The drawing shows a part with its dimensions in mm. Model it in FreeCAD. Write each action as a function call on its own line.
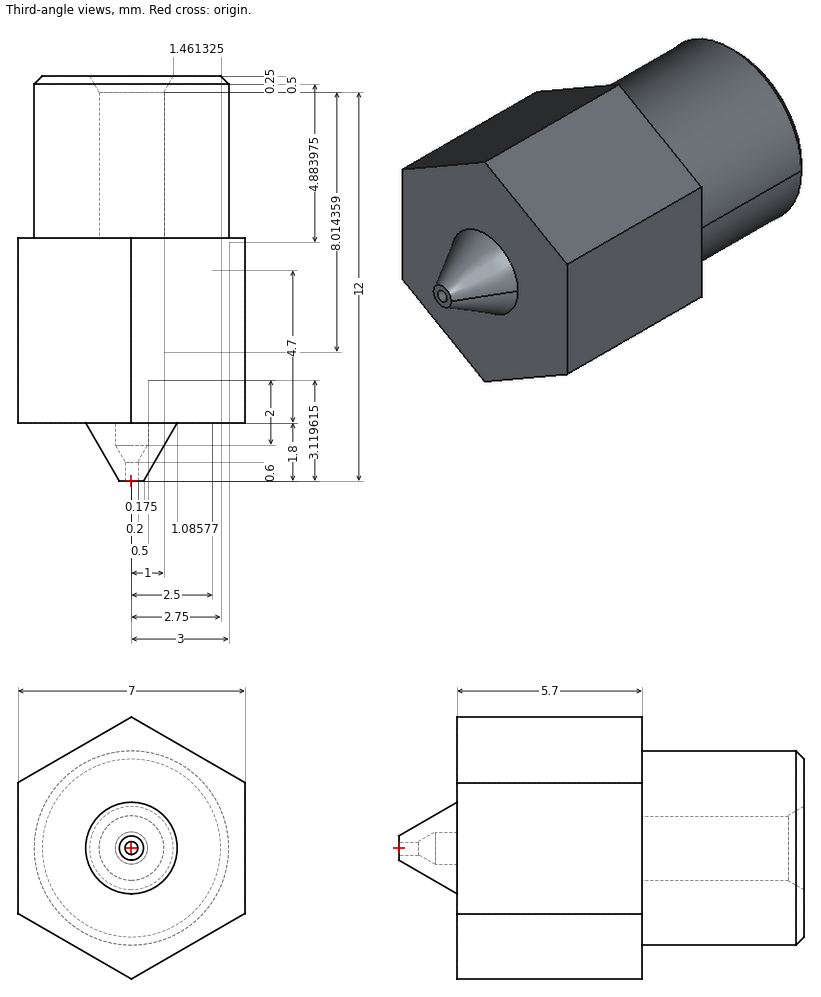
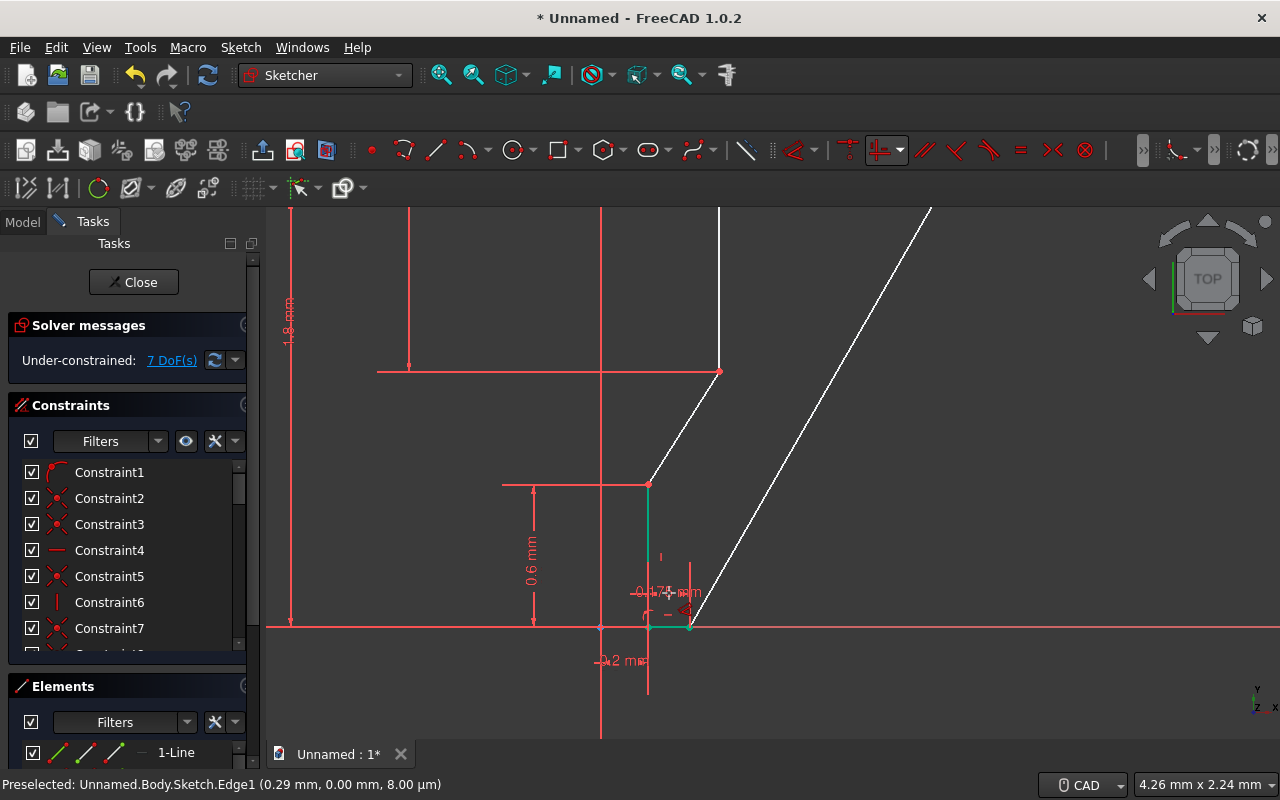
scroll(673, 639, down, 11)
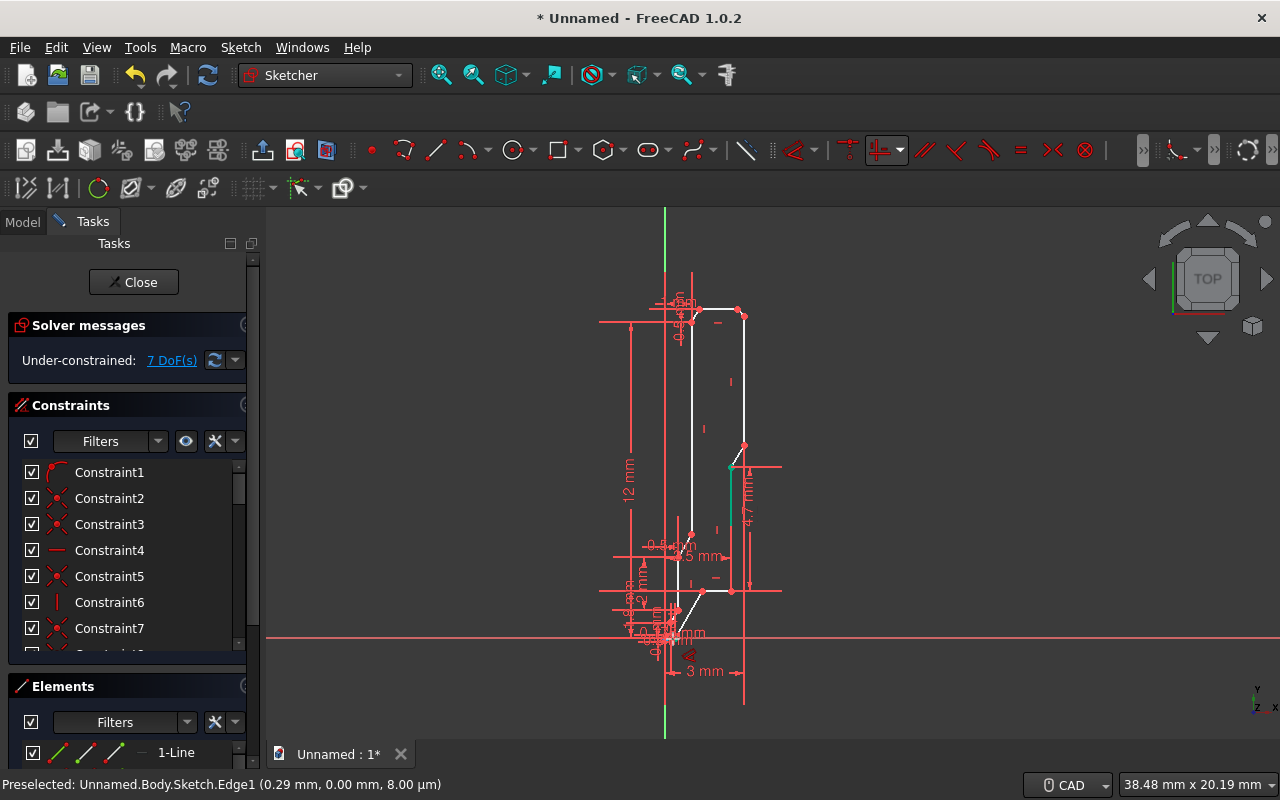
click(738, 309)
click(702, 275)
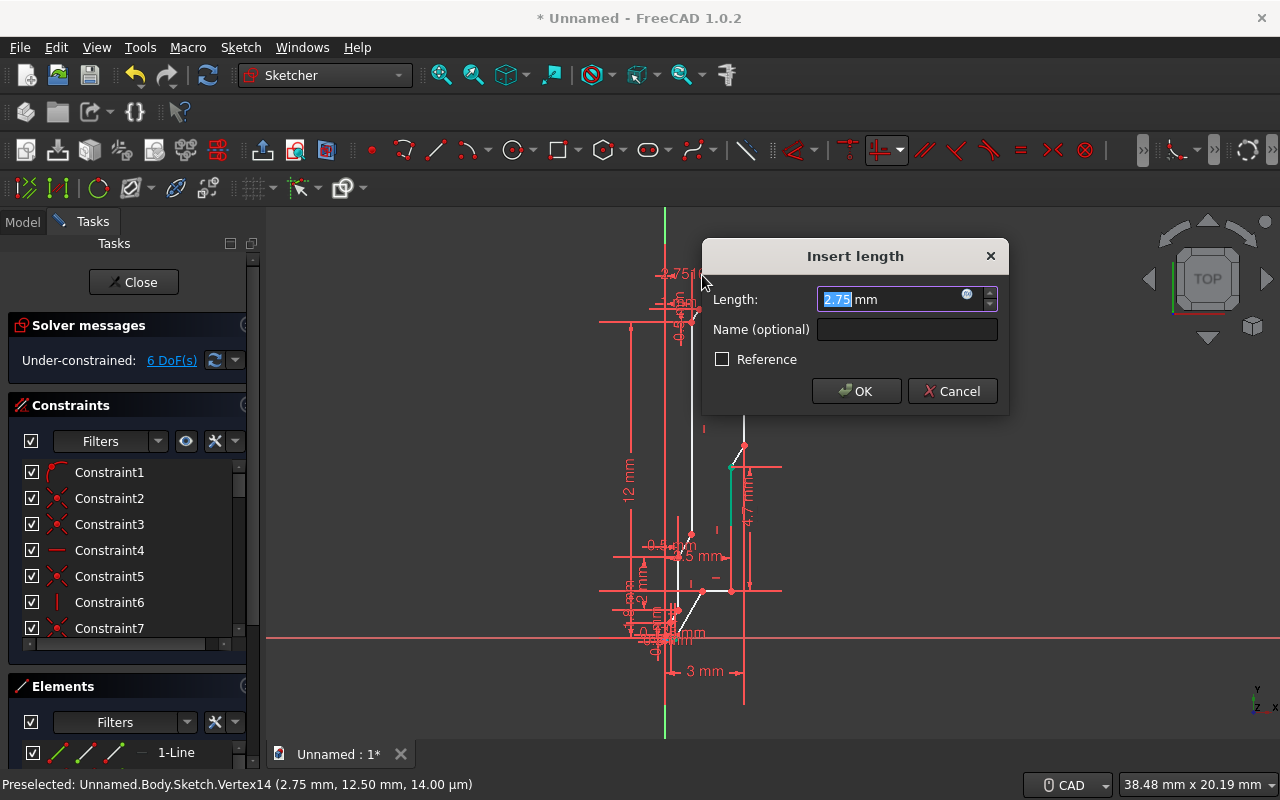
text(2.75)
key(Return)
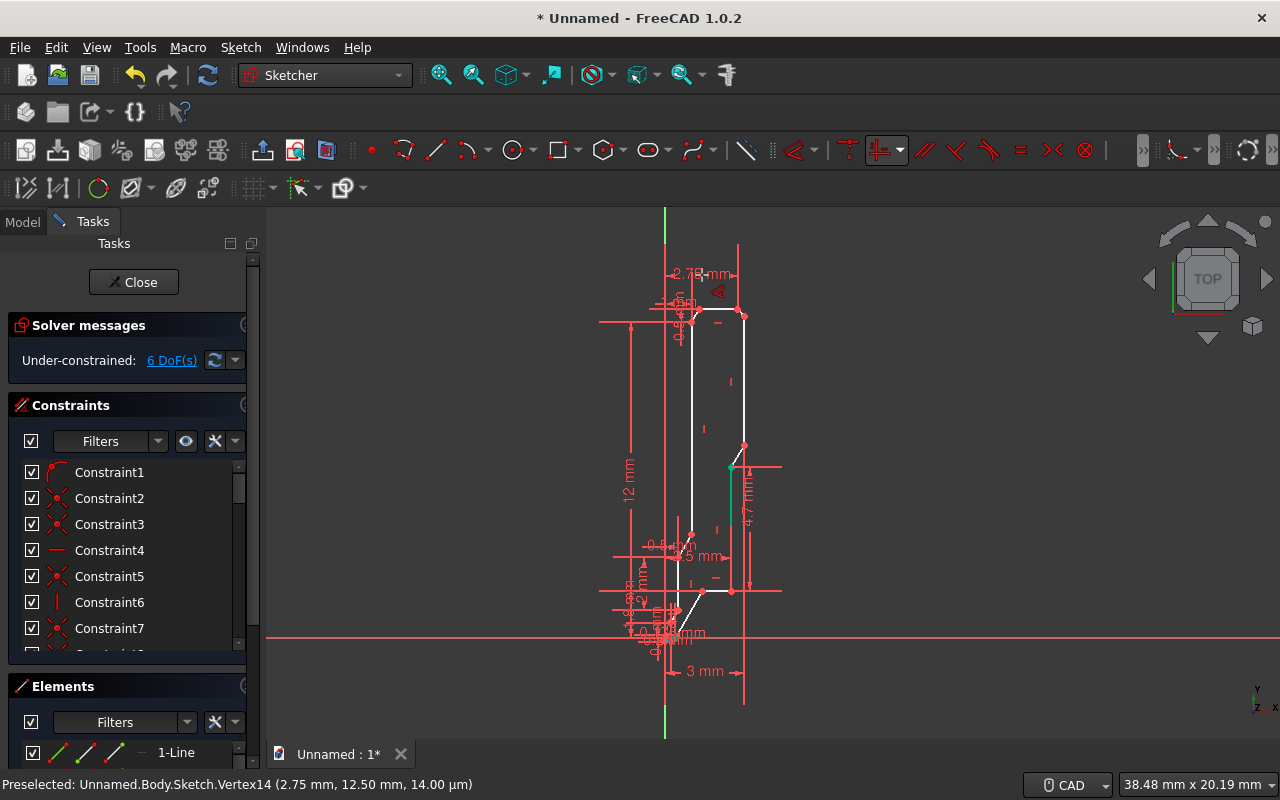
scroll(741, 313, up, 9)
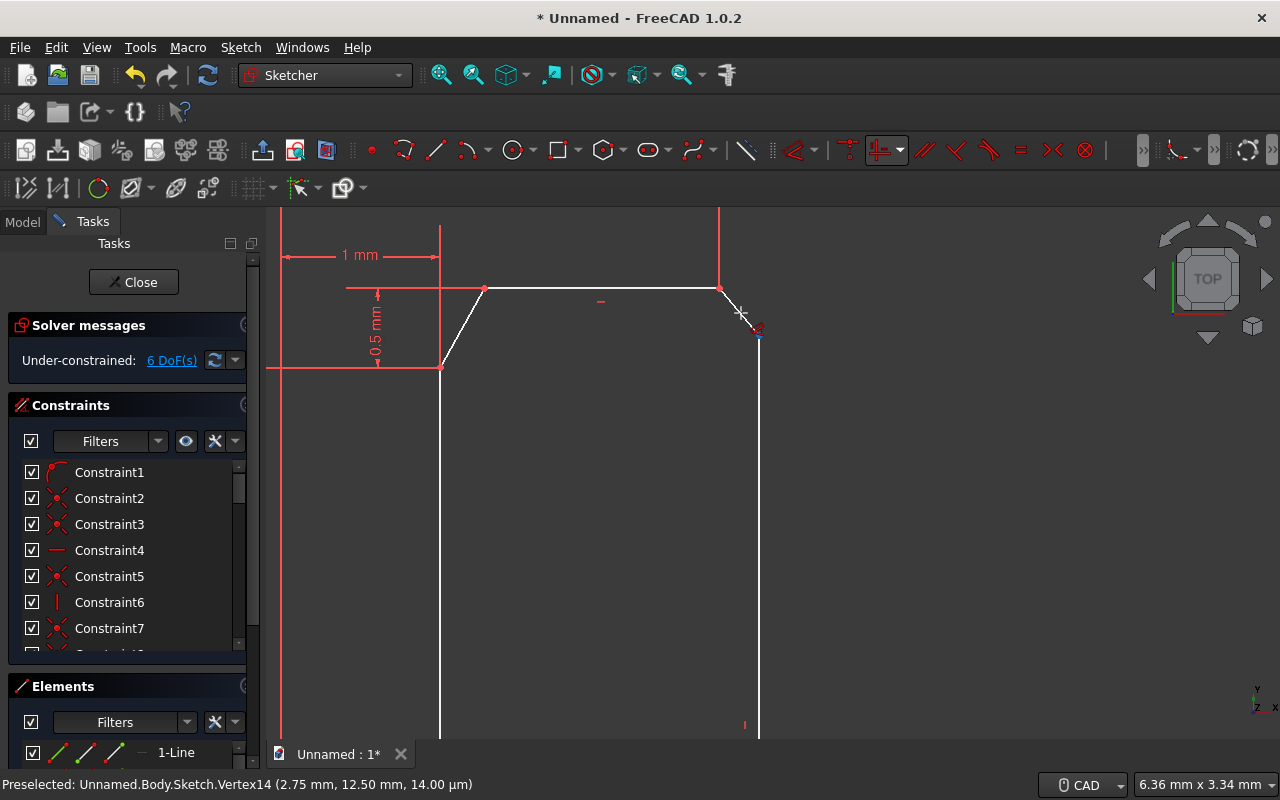
click(739, 312)
click(793, 312)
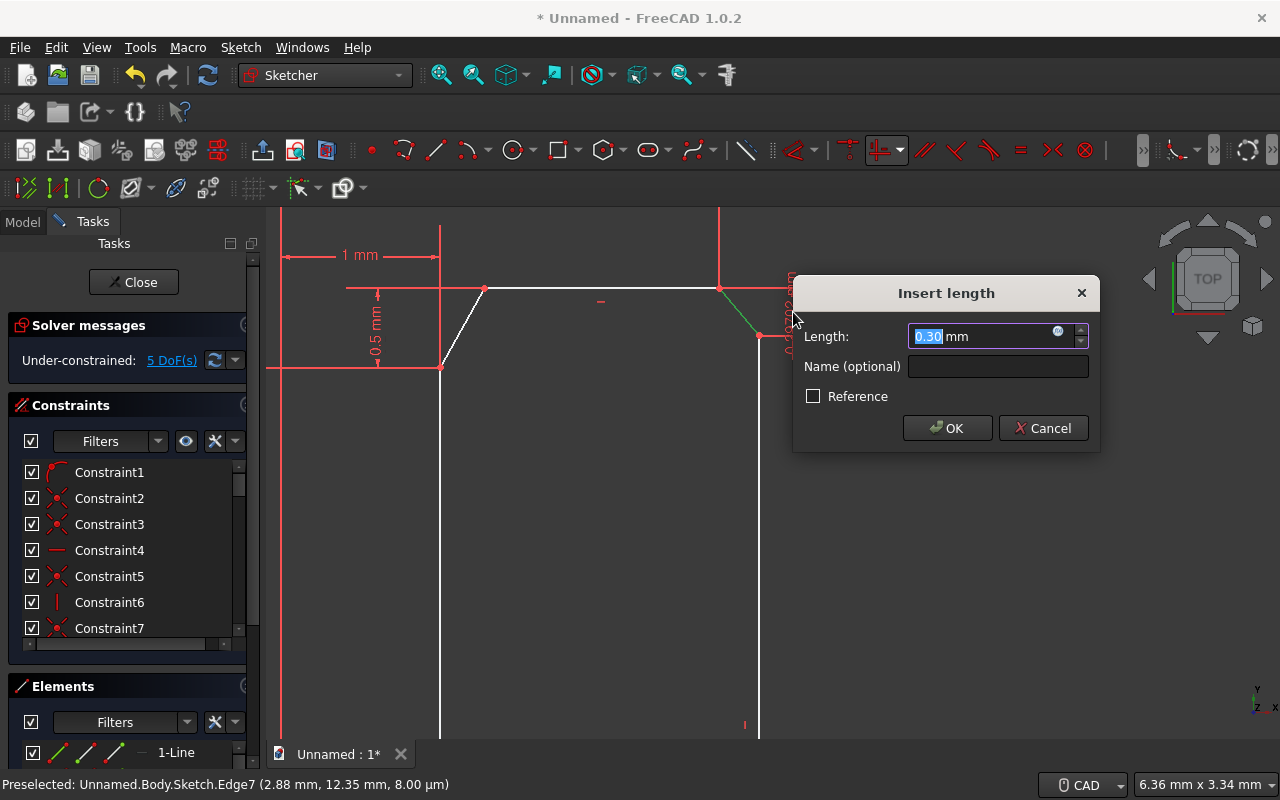
text(0.25)
key(Return)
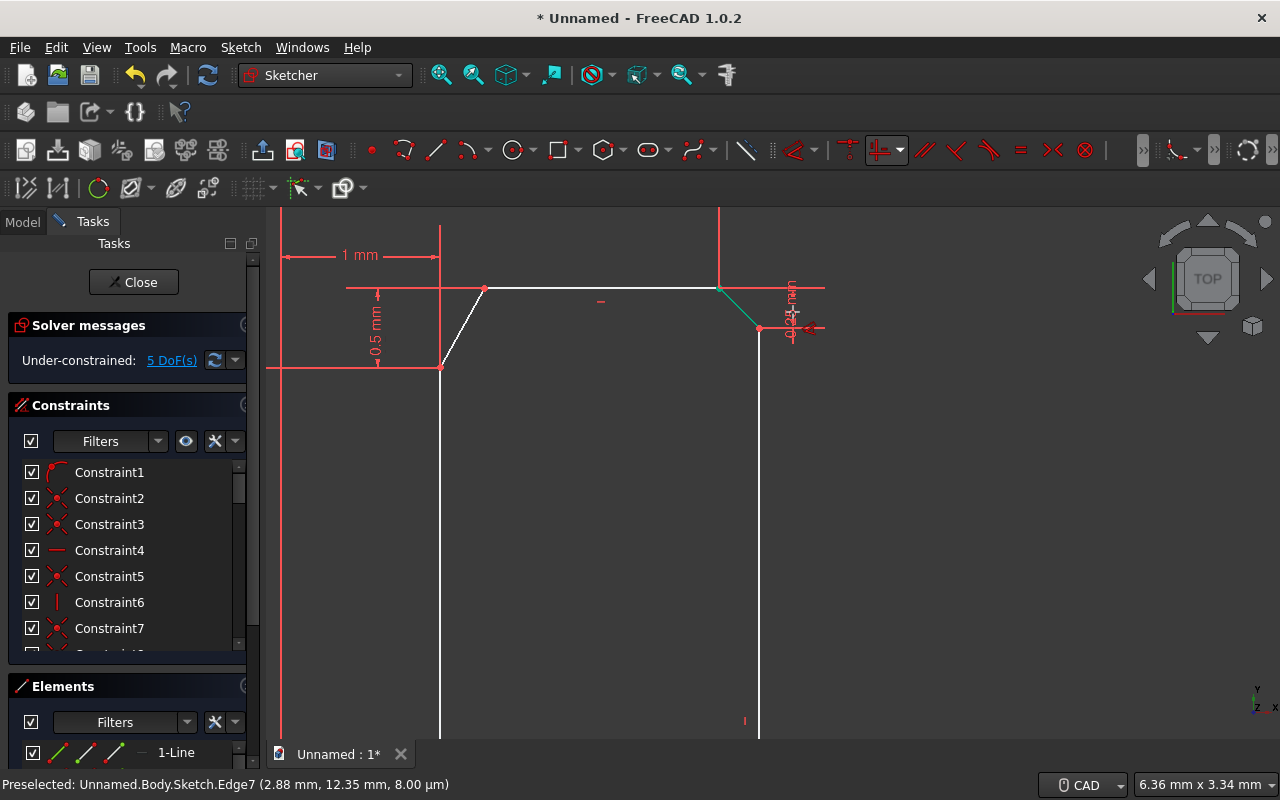
scroll(741, 312, down, 9)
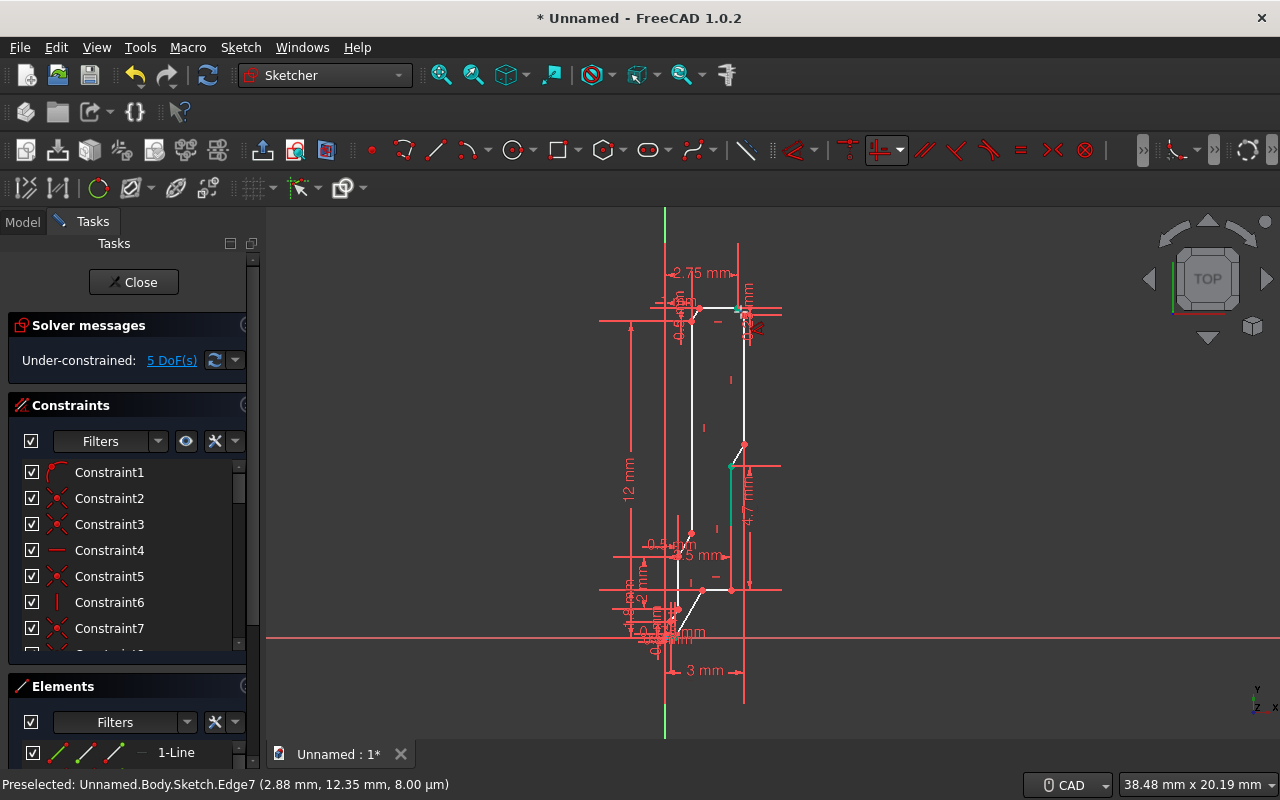
scroll(711, 590, up, 3)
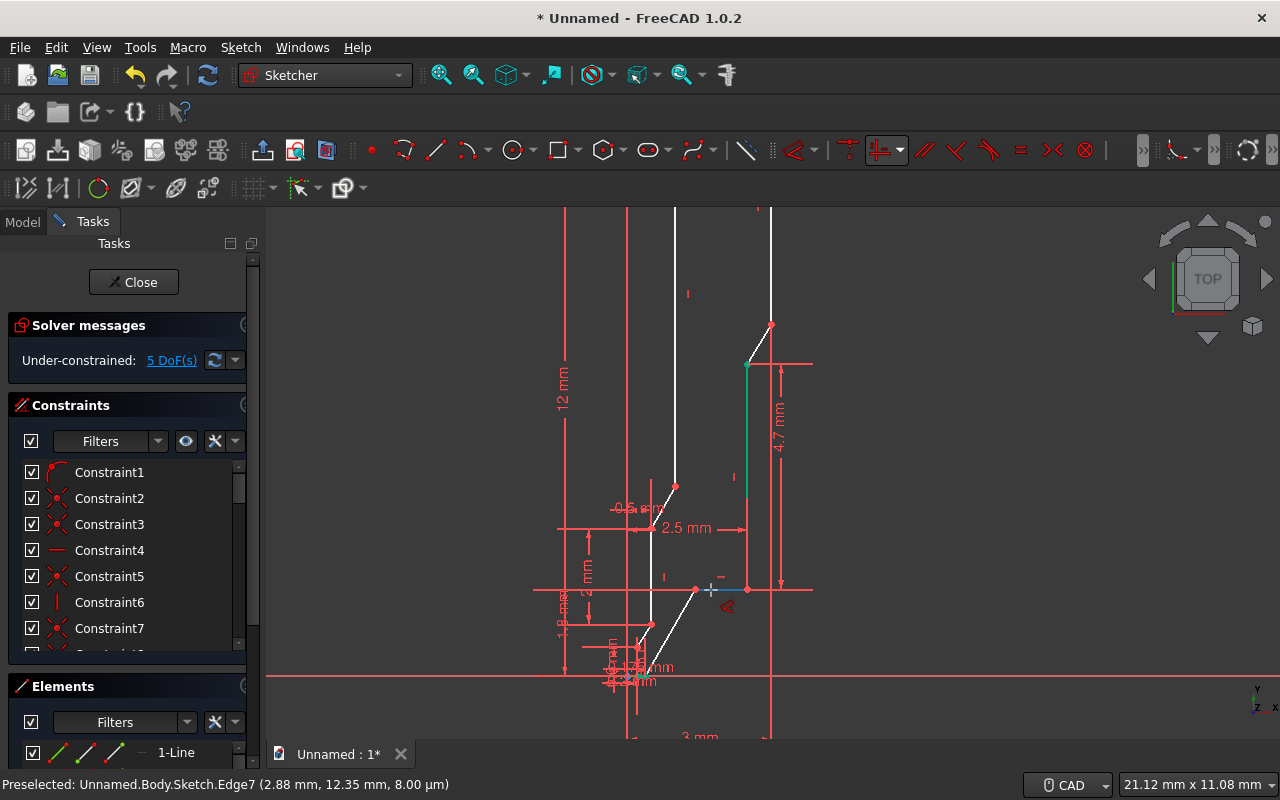
click(711, 590)
click(721, 624)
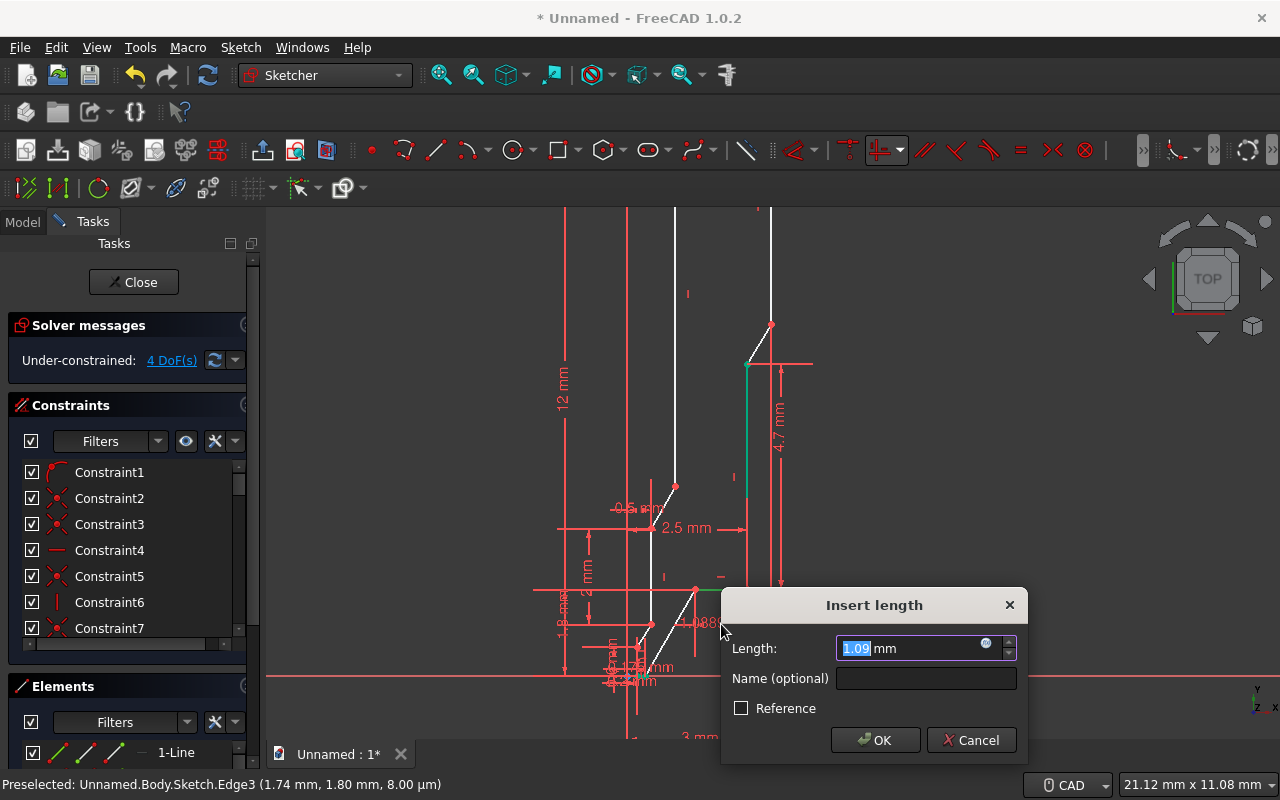
text(1.08577)
key(Return)